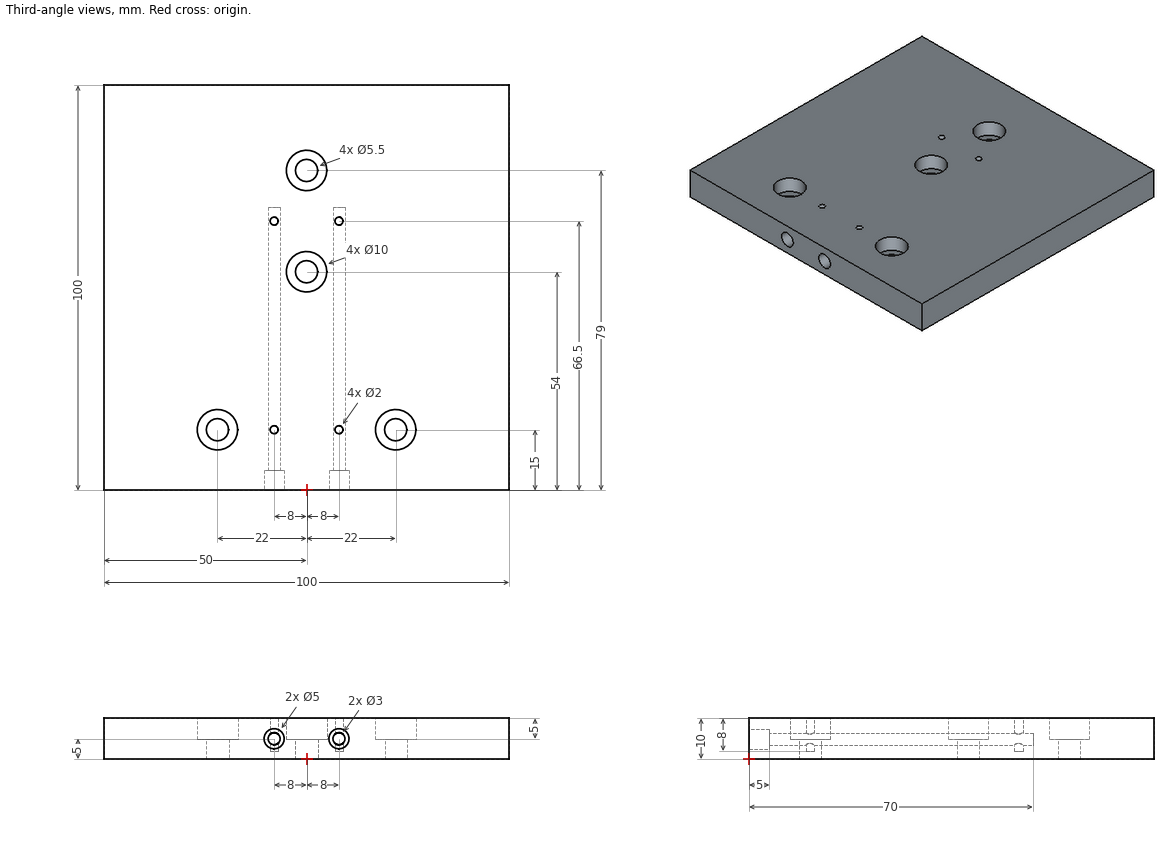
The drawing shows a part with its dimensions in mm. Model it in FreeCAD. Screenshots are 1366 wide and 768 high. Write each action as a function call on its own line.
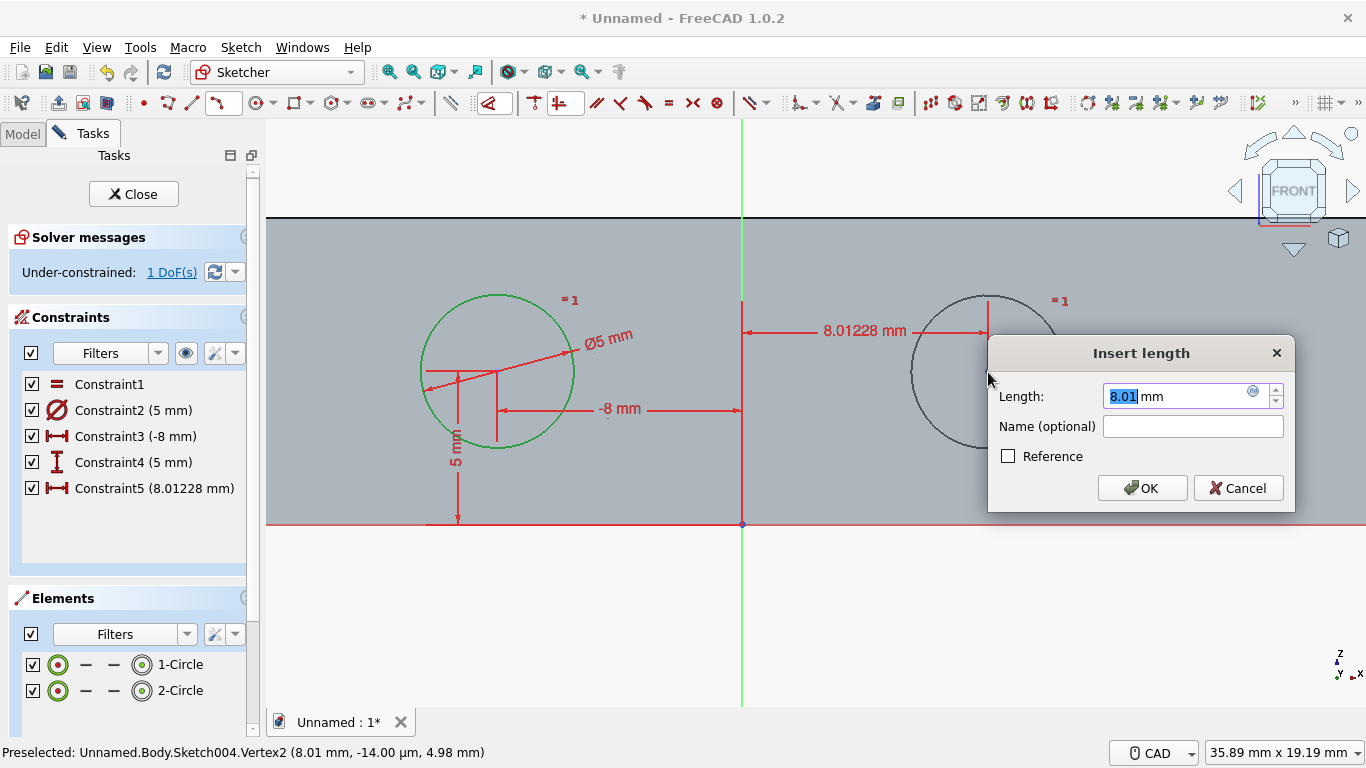
text(8)
key(Return)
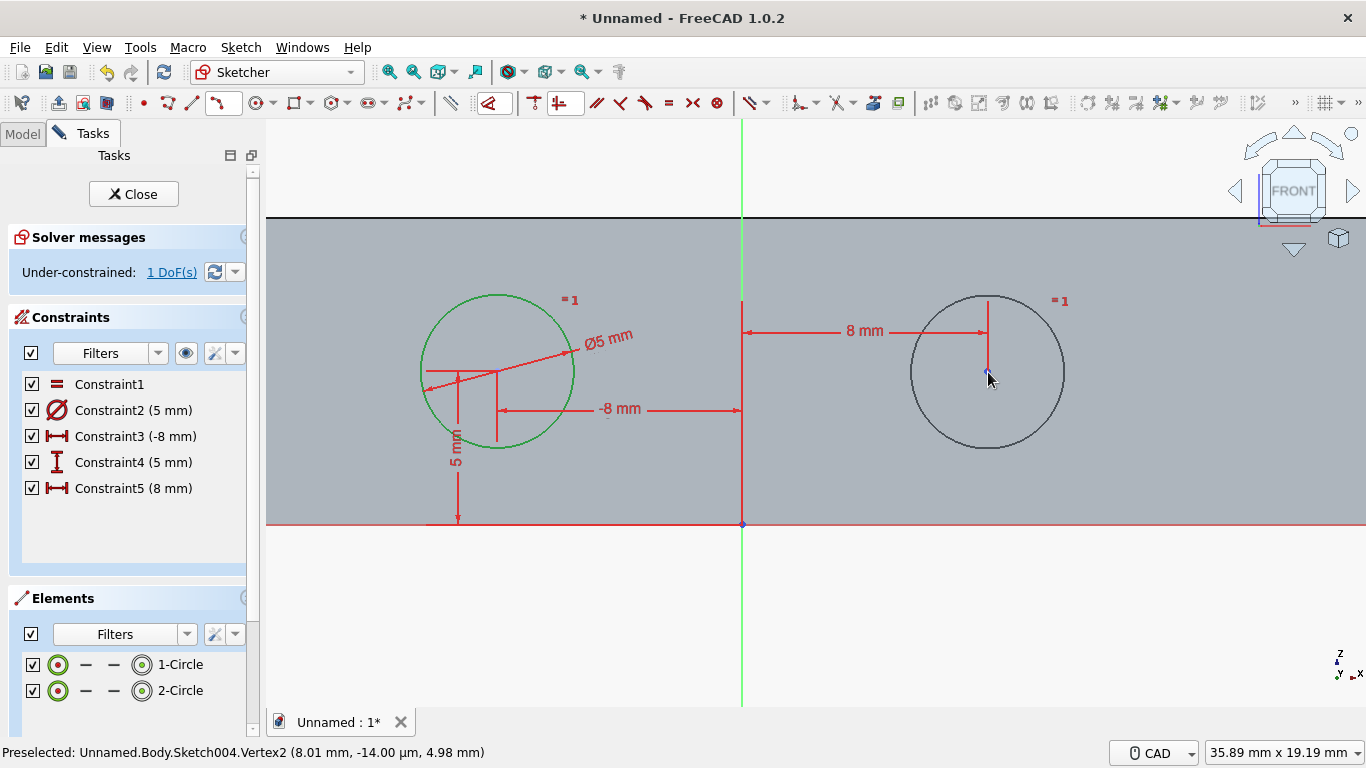
click(988, 372)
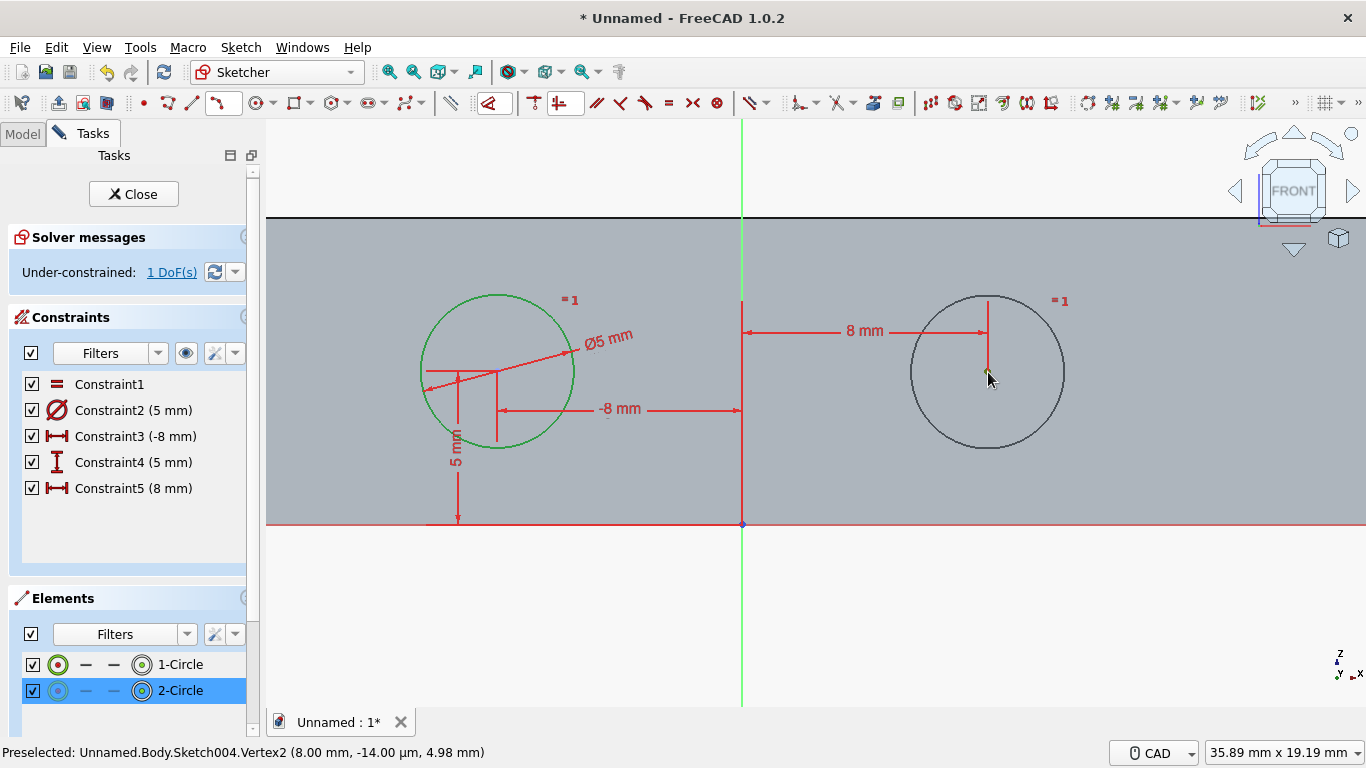
click(506, 104)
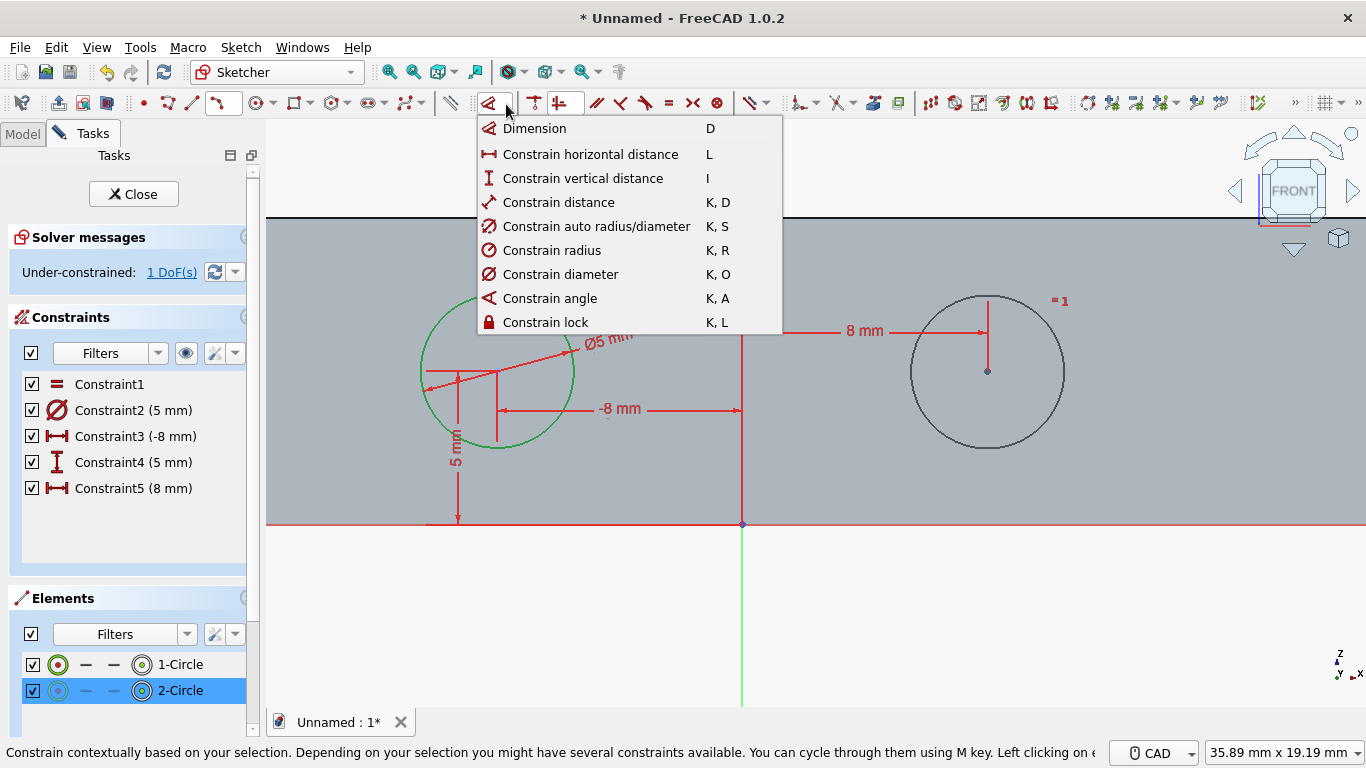
click(630, 178)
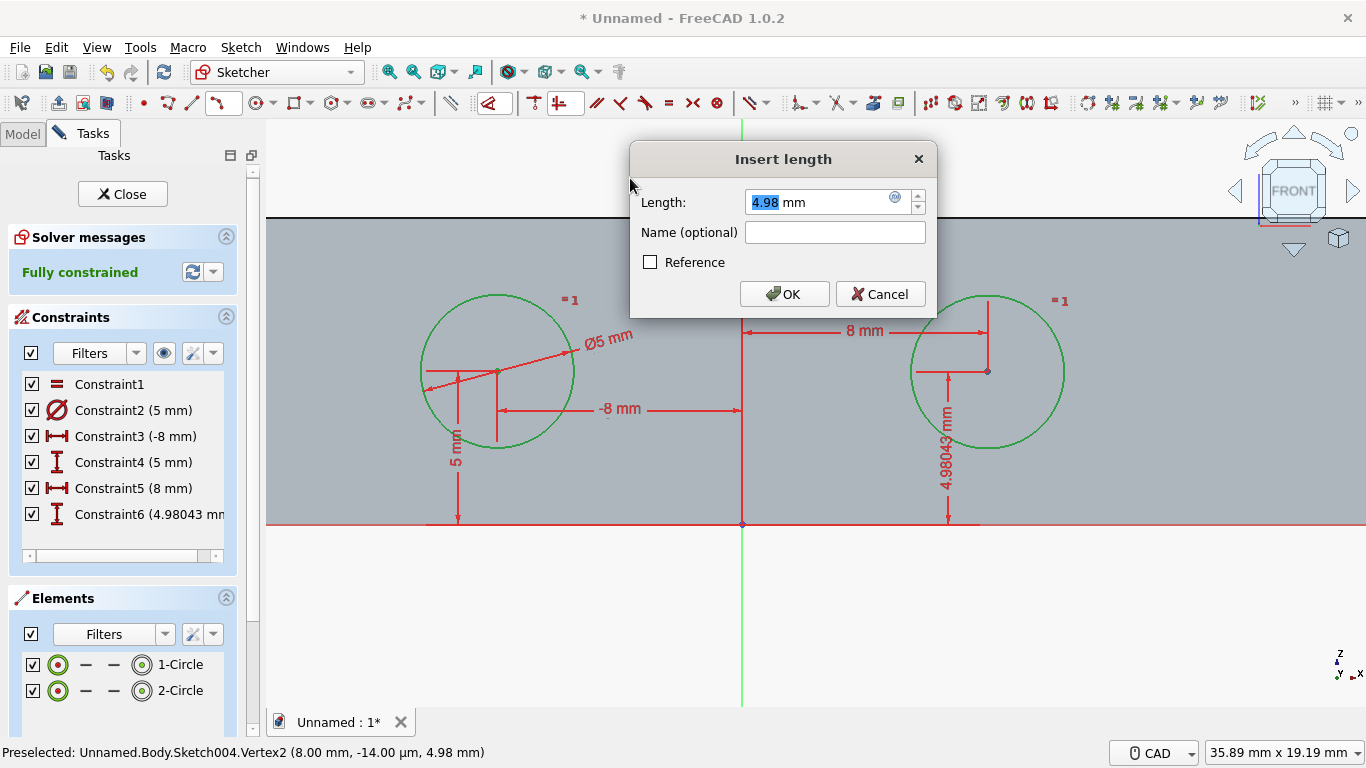
text(5)
key(Return)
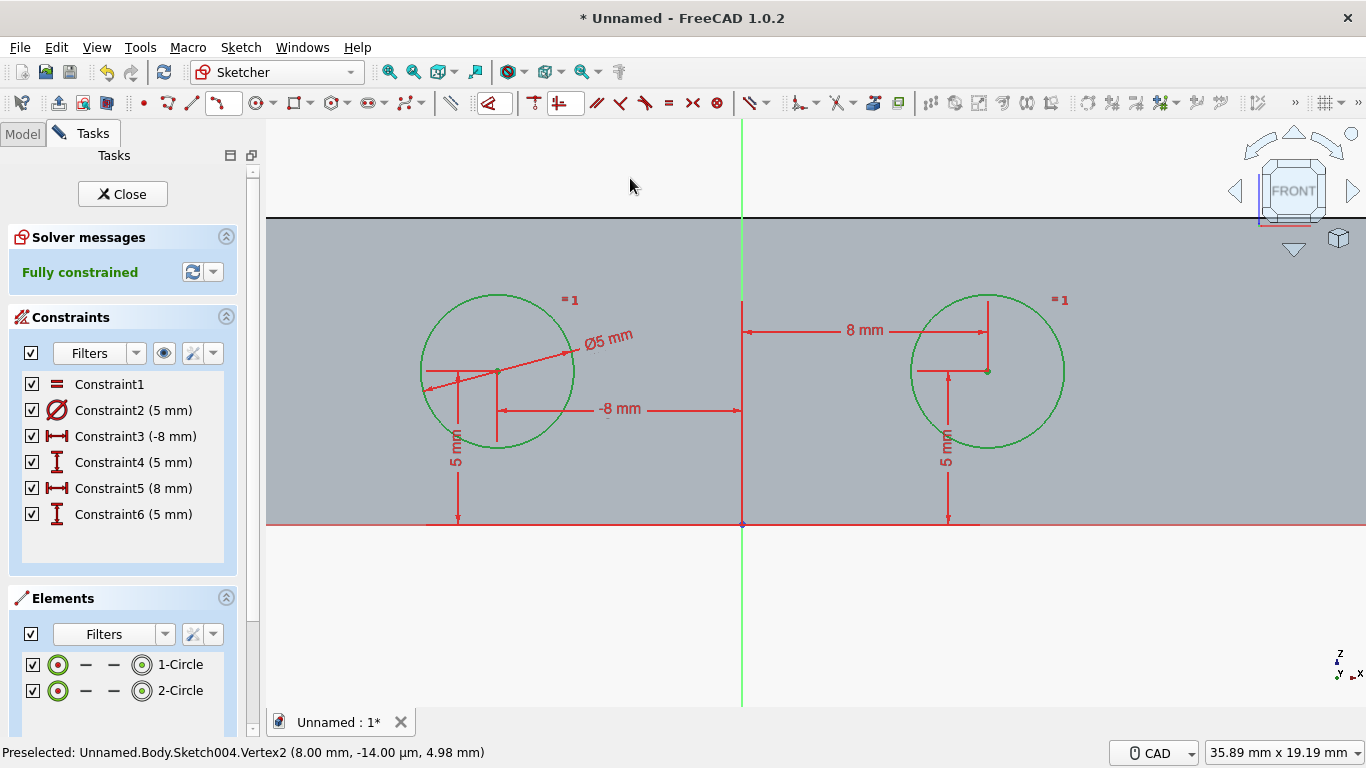
click(123, 194)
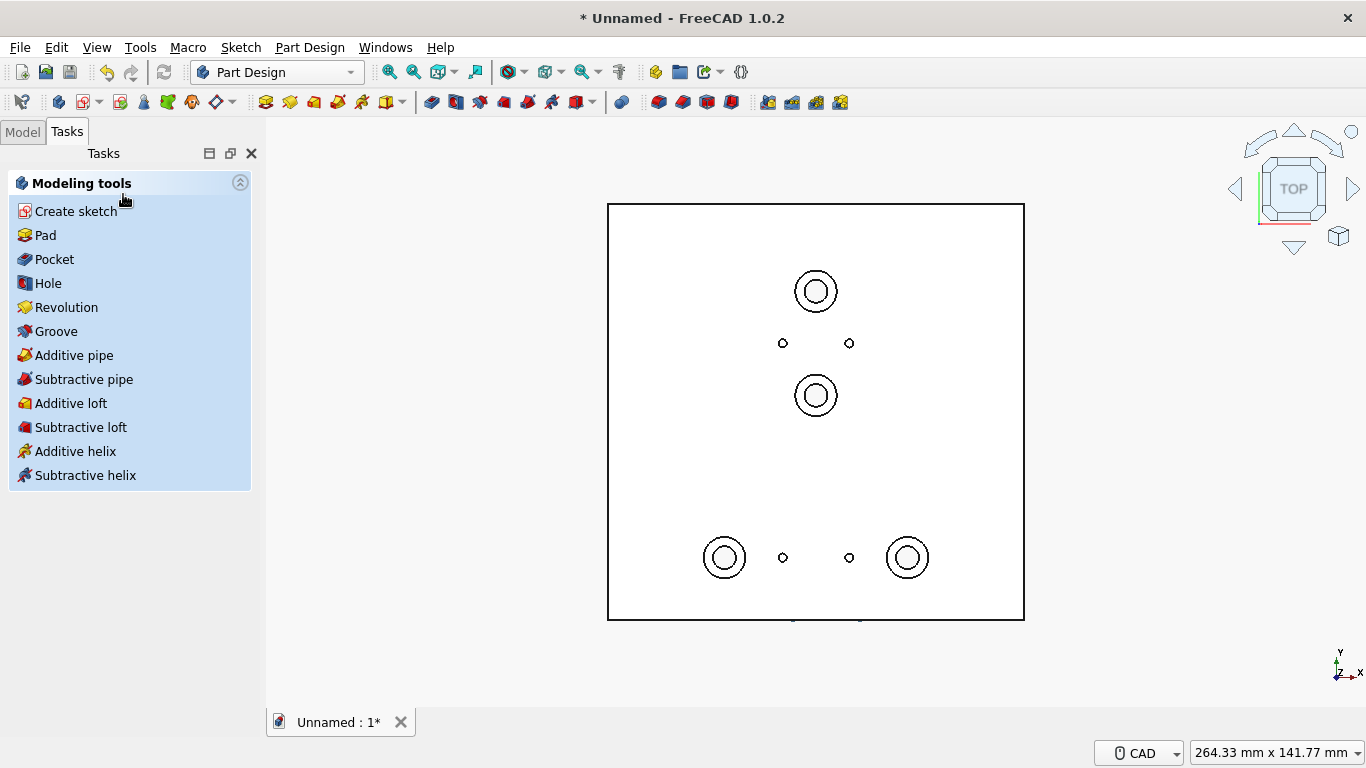
click(432, 102)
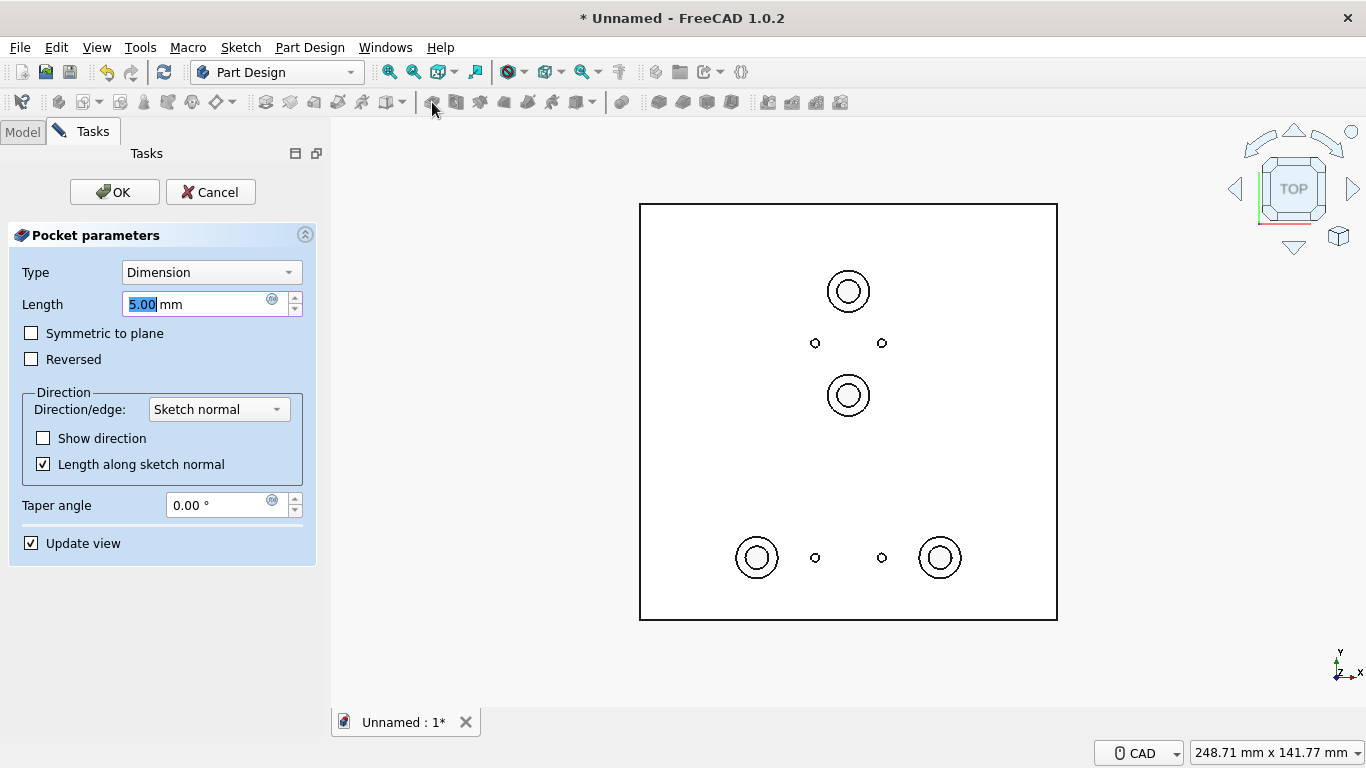
text(5)
key(Tab)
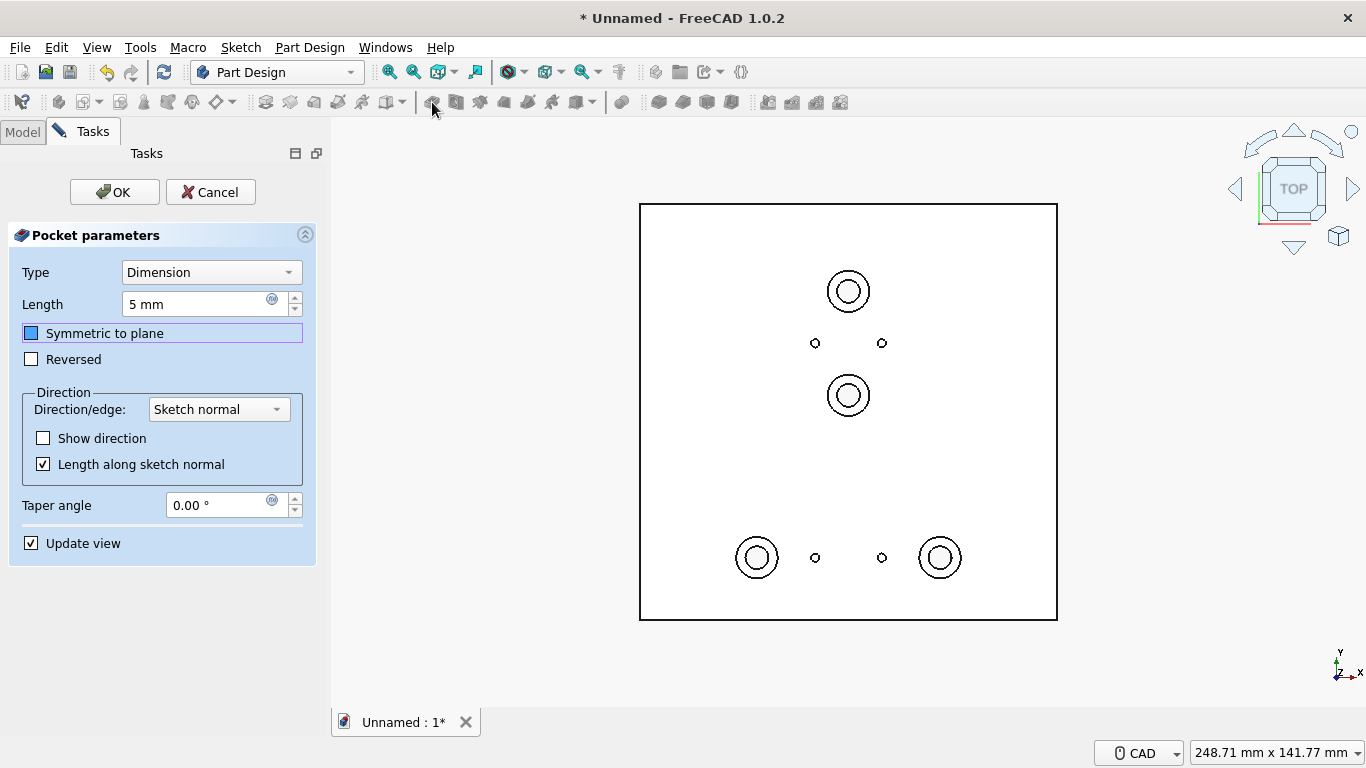
click(115, 192)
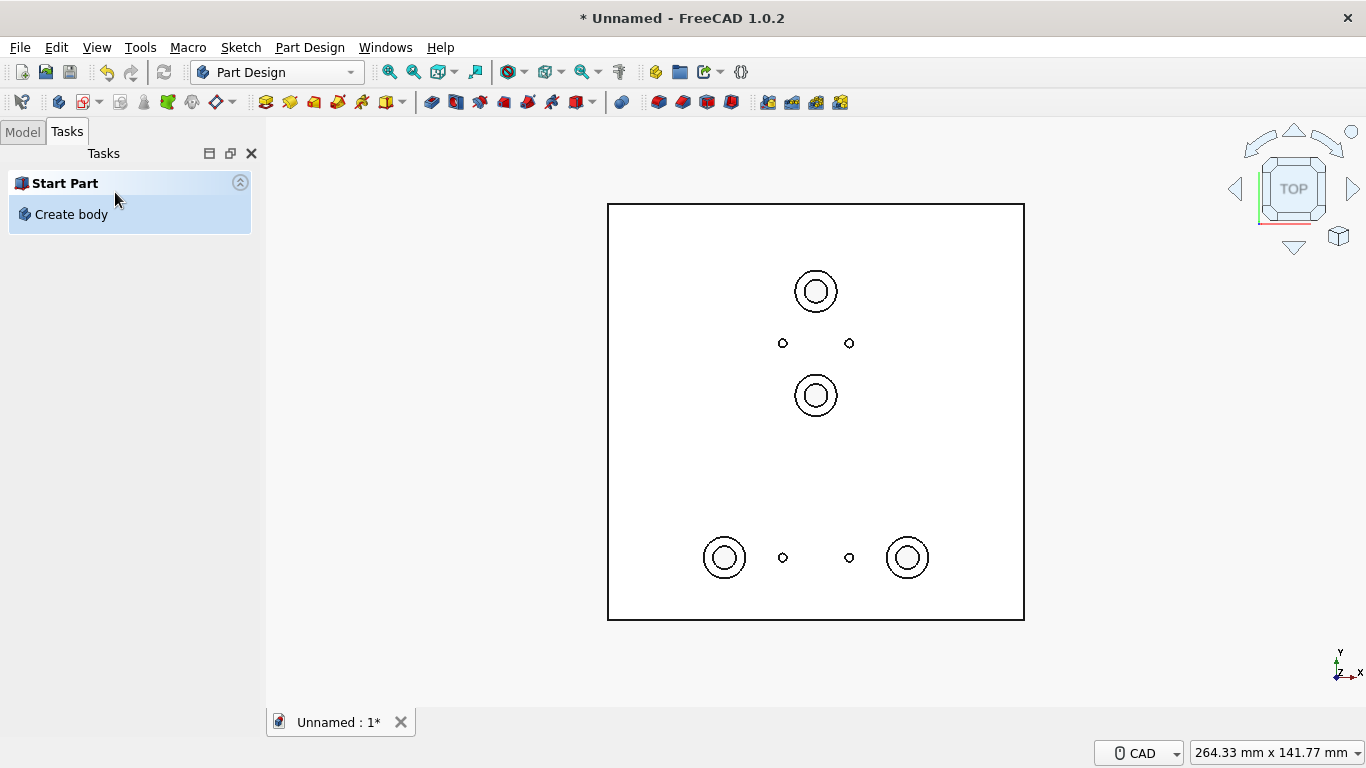
click(84, 102)